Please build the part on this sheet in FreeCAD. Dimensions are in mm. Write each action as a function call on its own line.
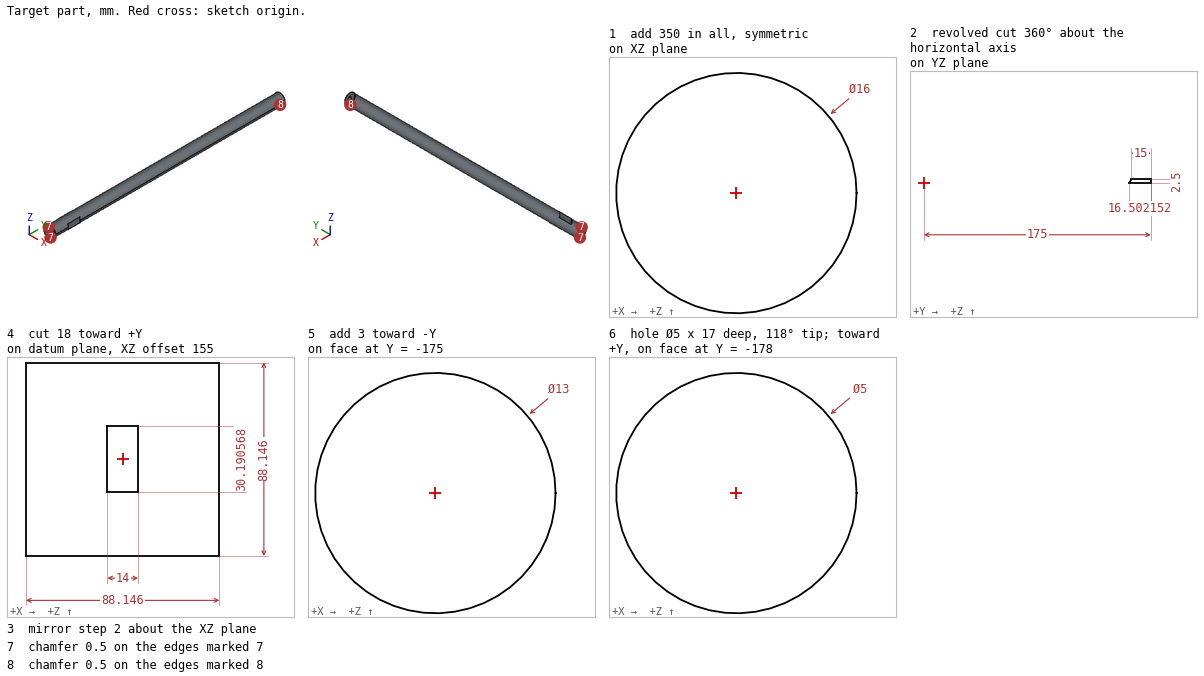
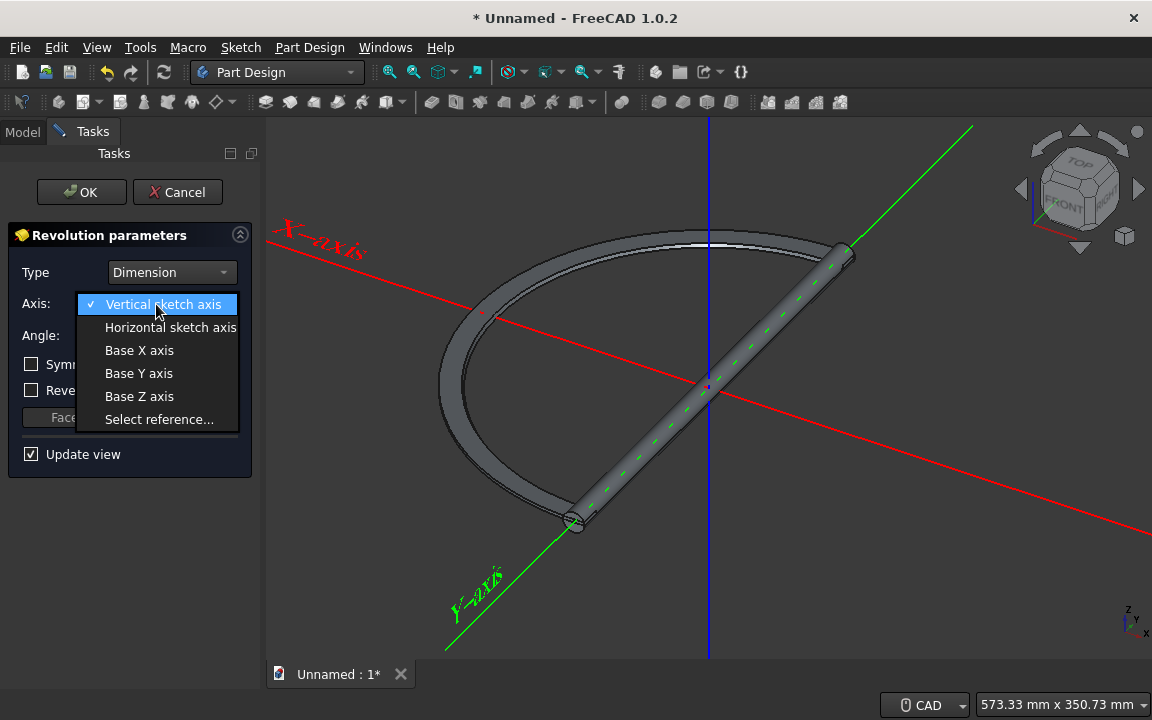
click(156, 328)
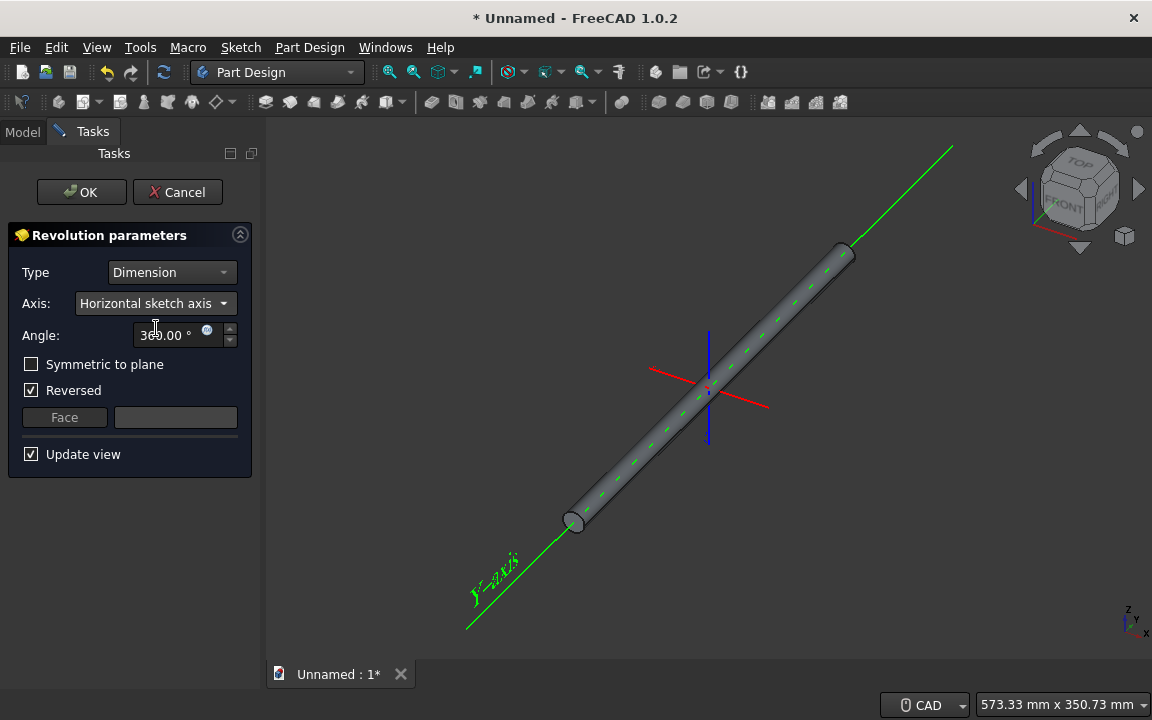
click(82, 192)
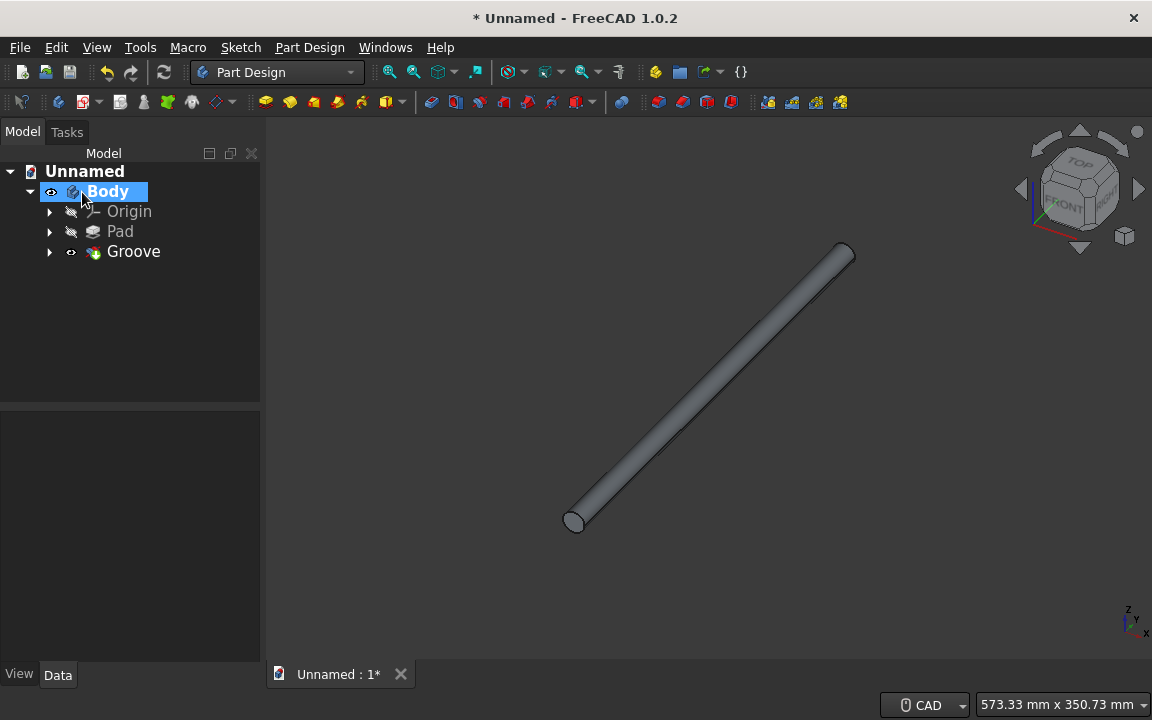
click(116, 252)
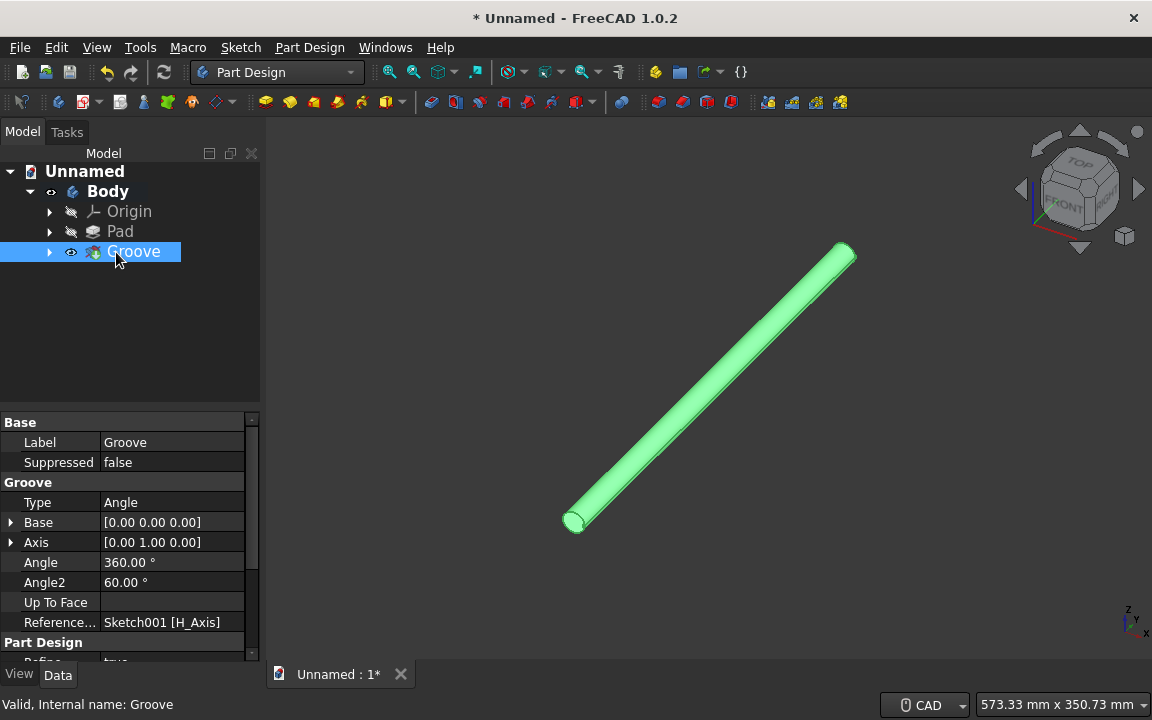
click(768, 102)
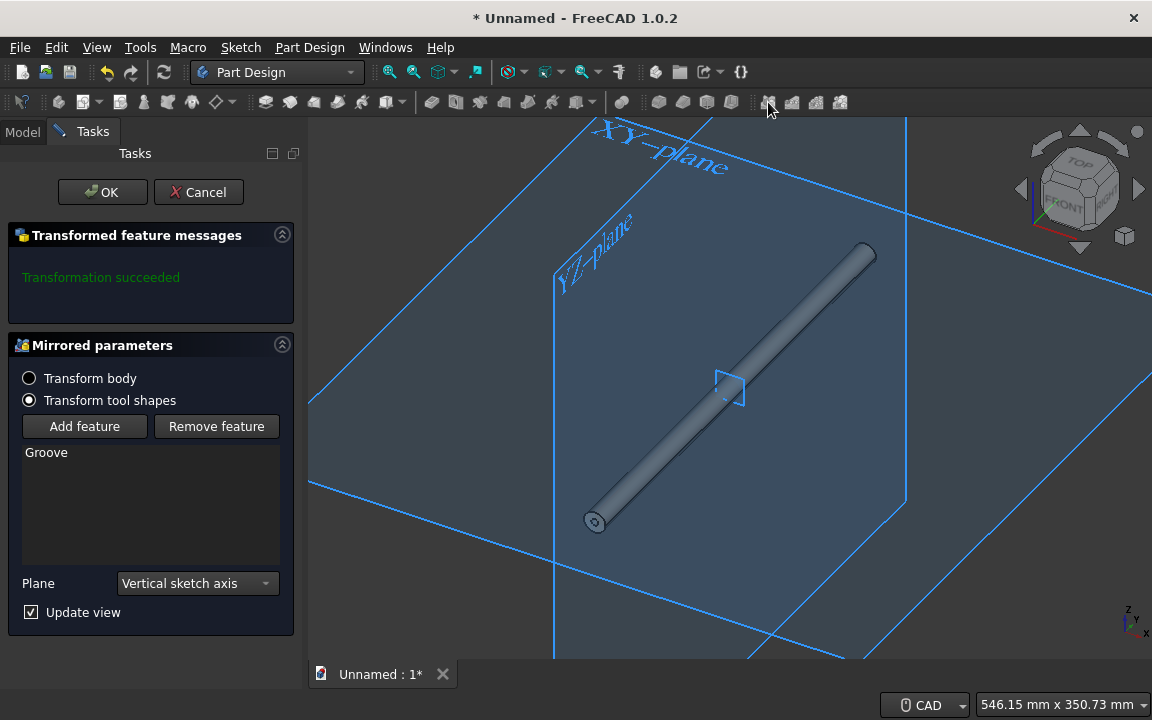
click(198, 584)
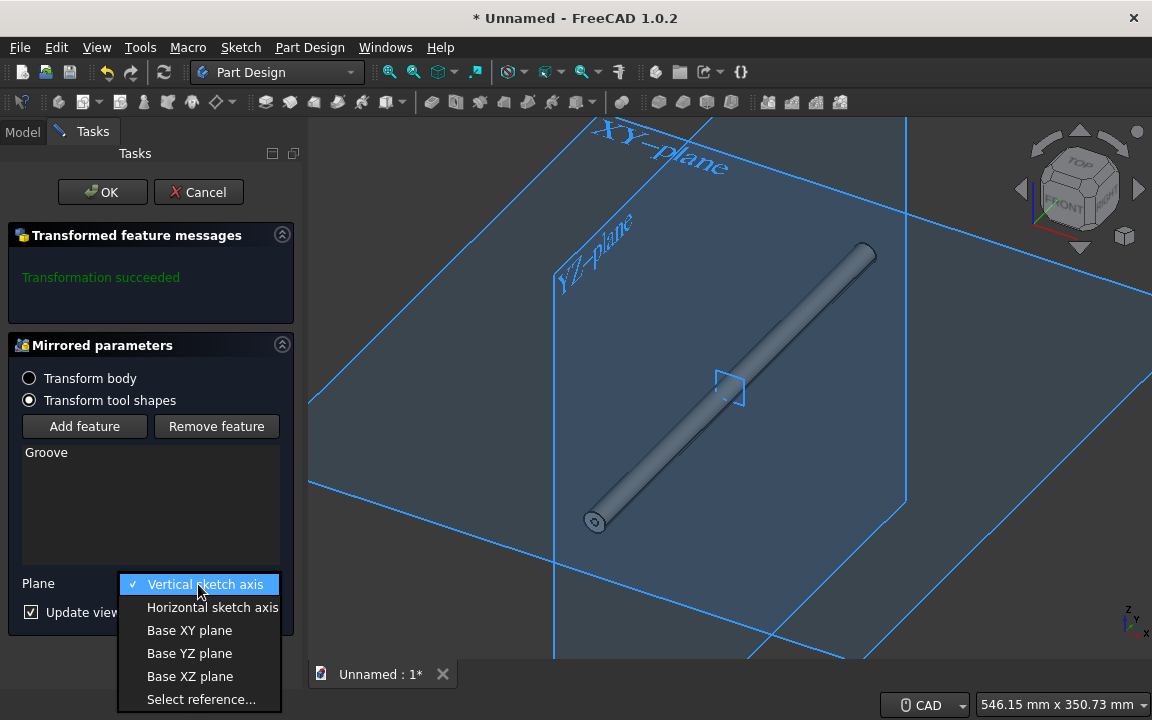
click(198, 676)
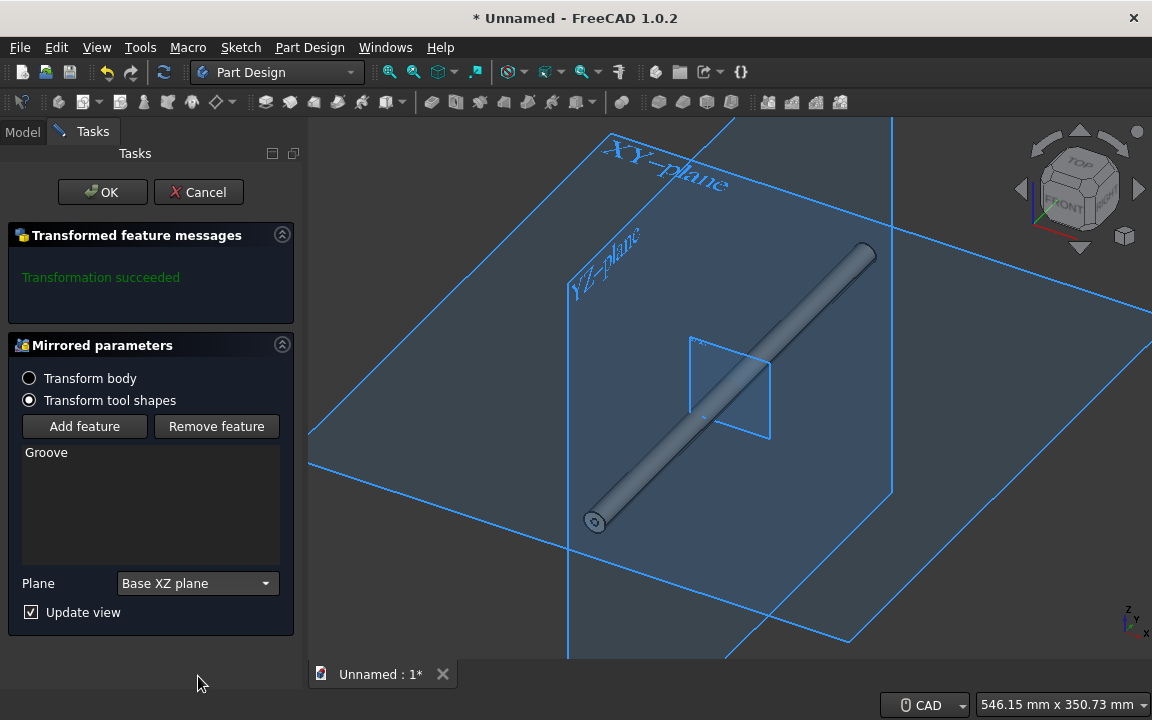
click(103, 192)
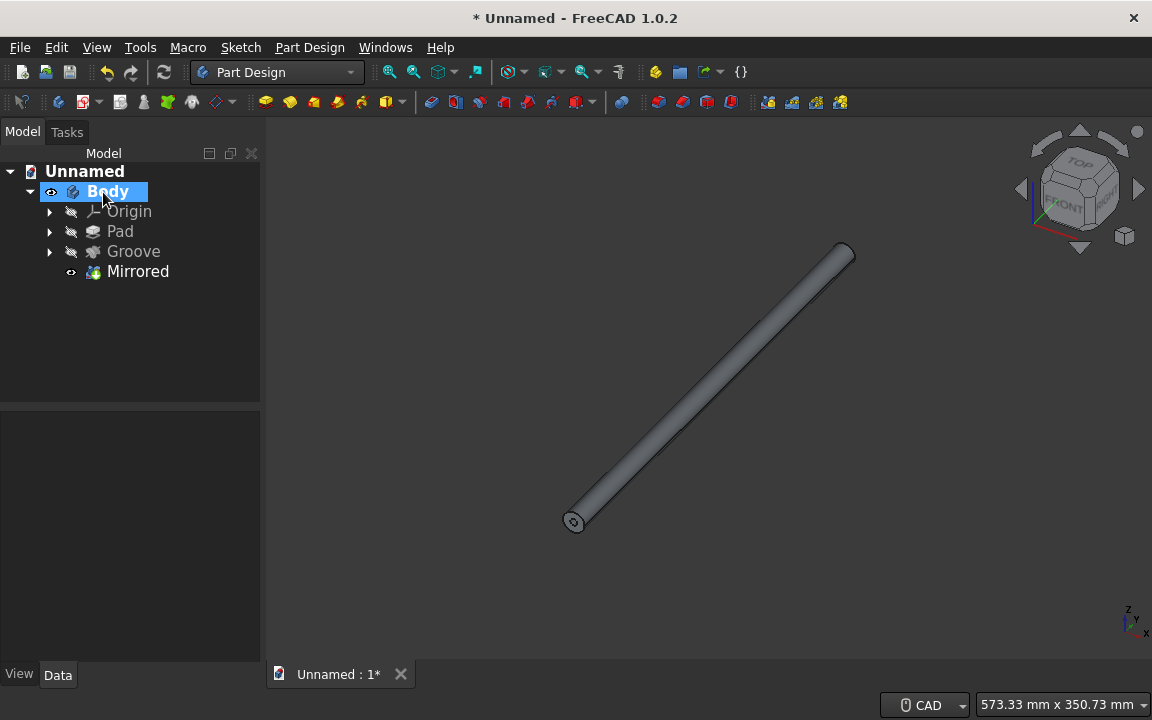
click(50, 212)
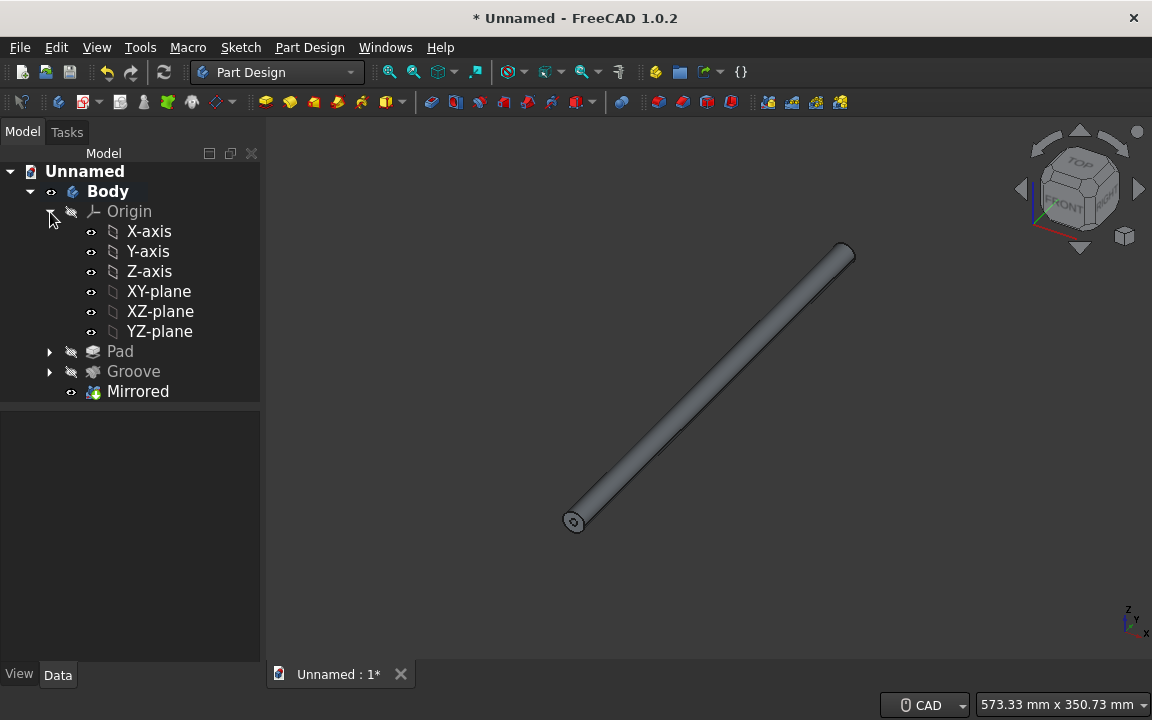
click(136, 312)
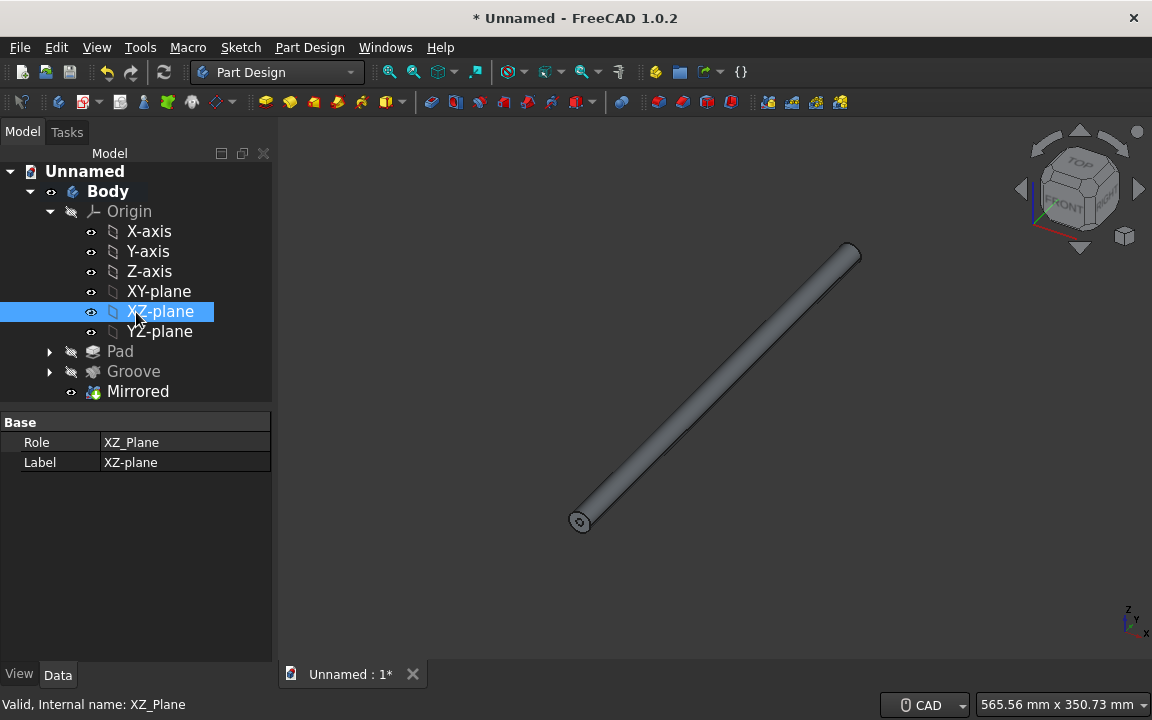
click(216, 102)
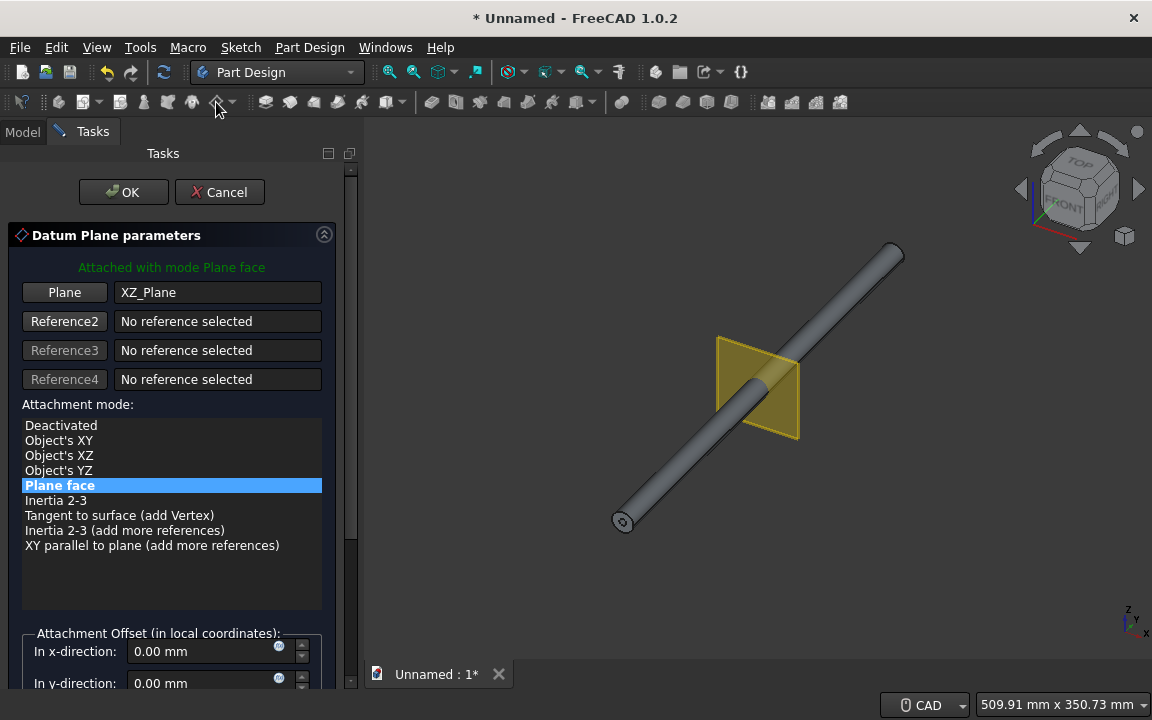
scroll(351, 426, down, 2)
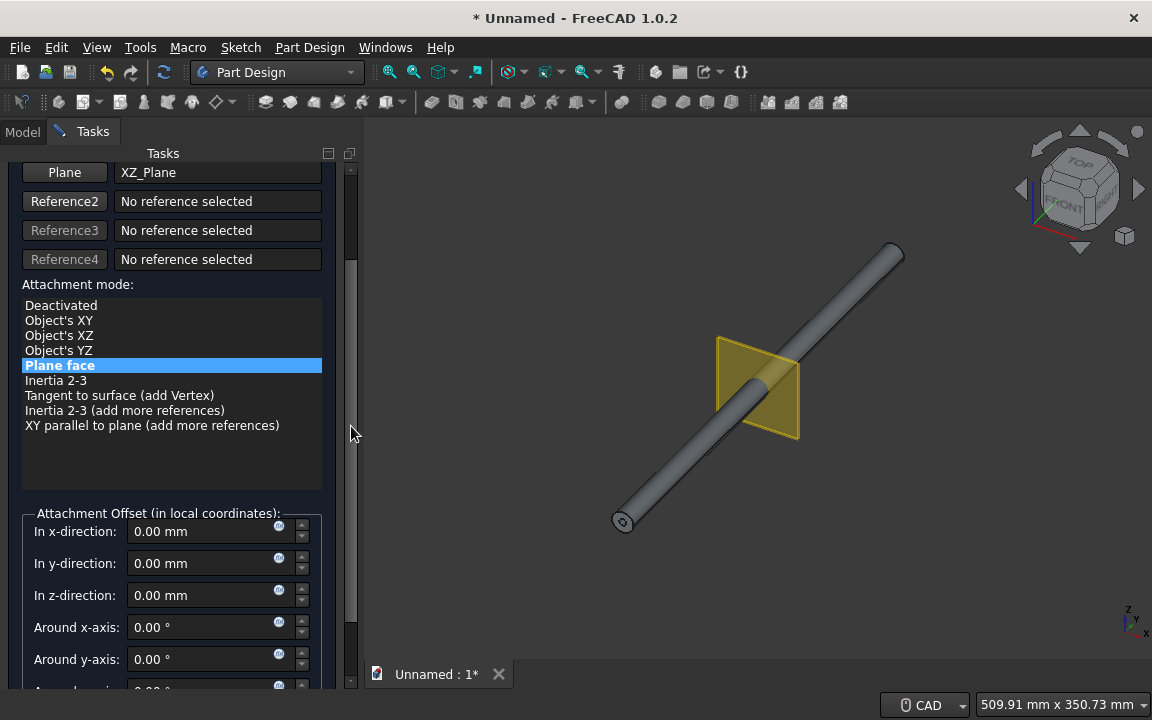
triple_click(210, 595)